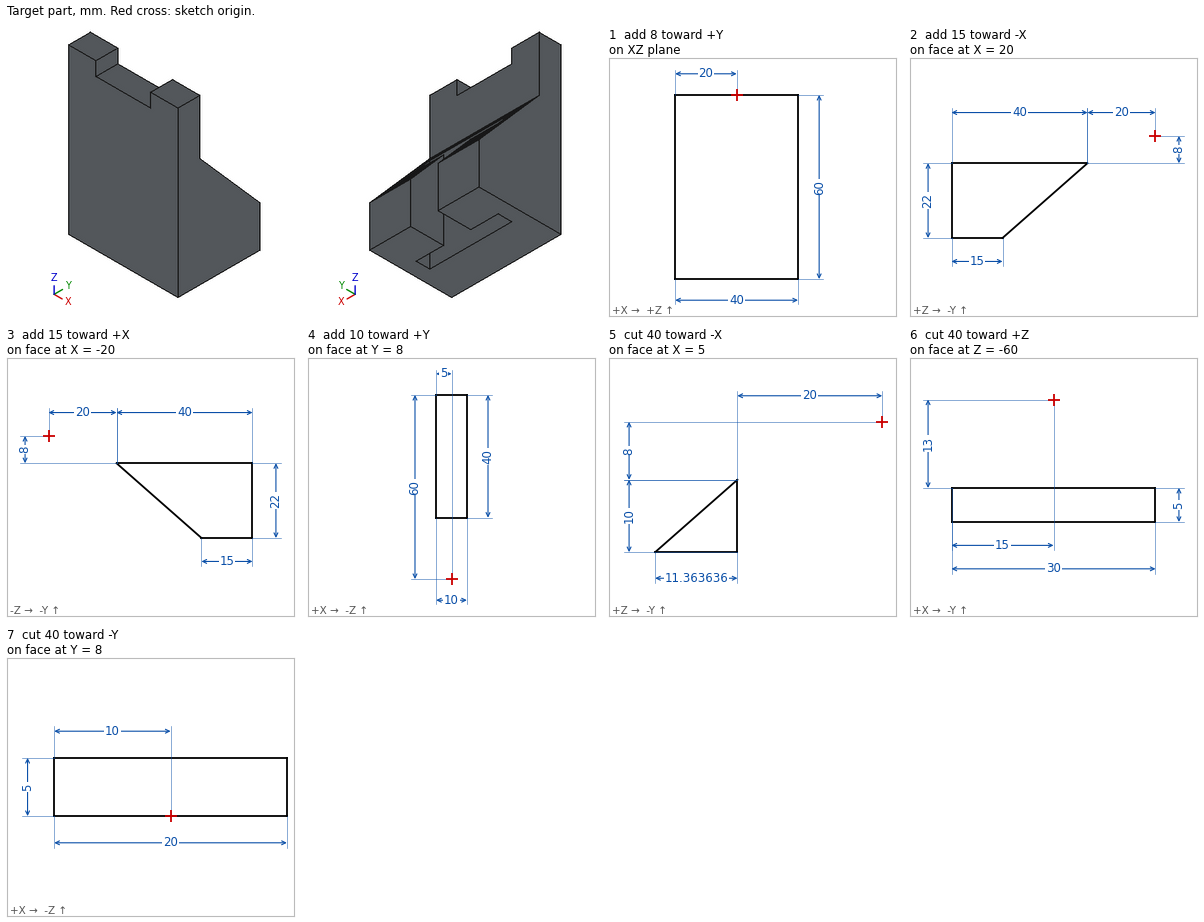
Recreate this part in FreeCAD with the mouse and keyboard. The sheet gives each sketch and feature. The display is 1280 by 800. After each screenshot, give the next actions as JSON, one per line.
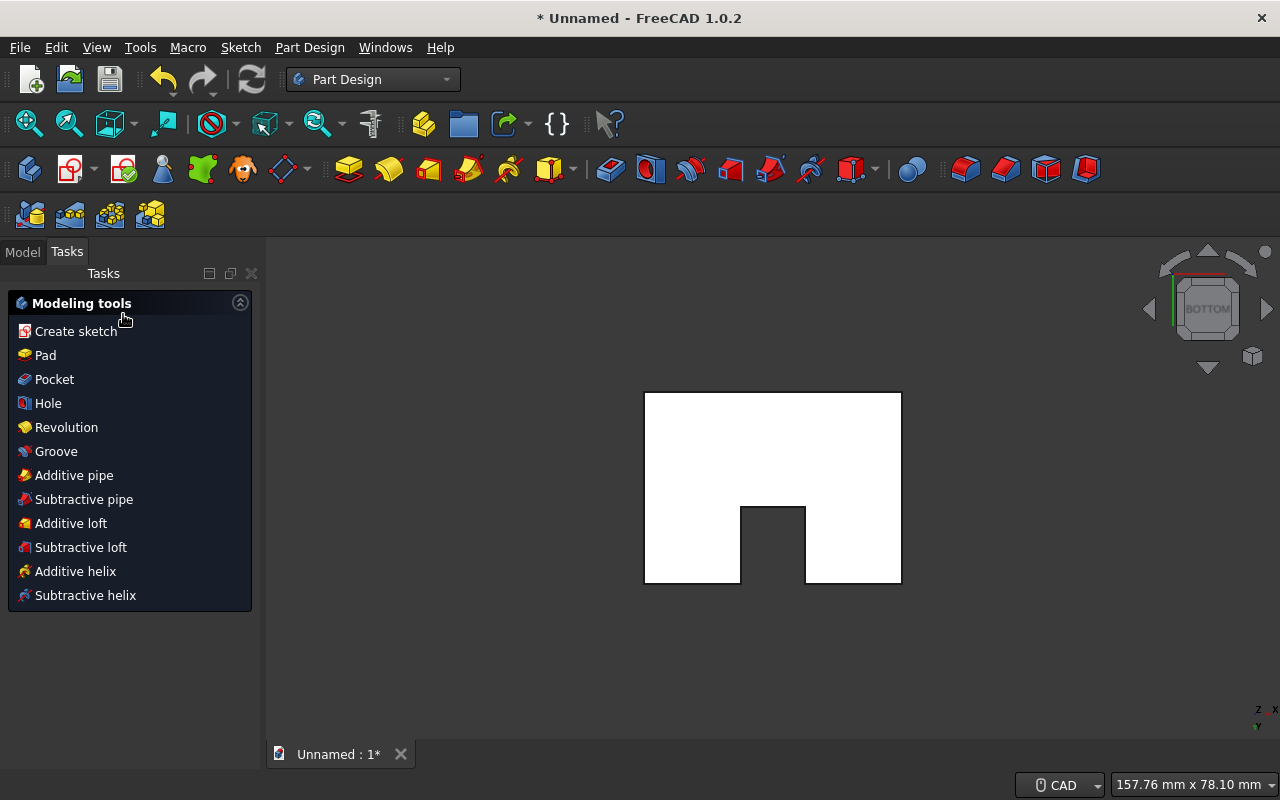
{"action": "left_click", "coordinate": [612, 170]}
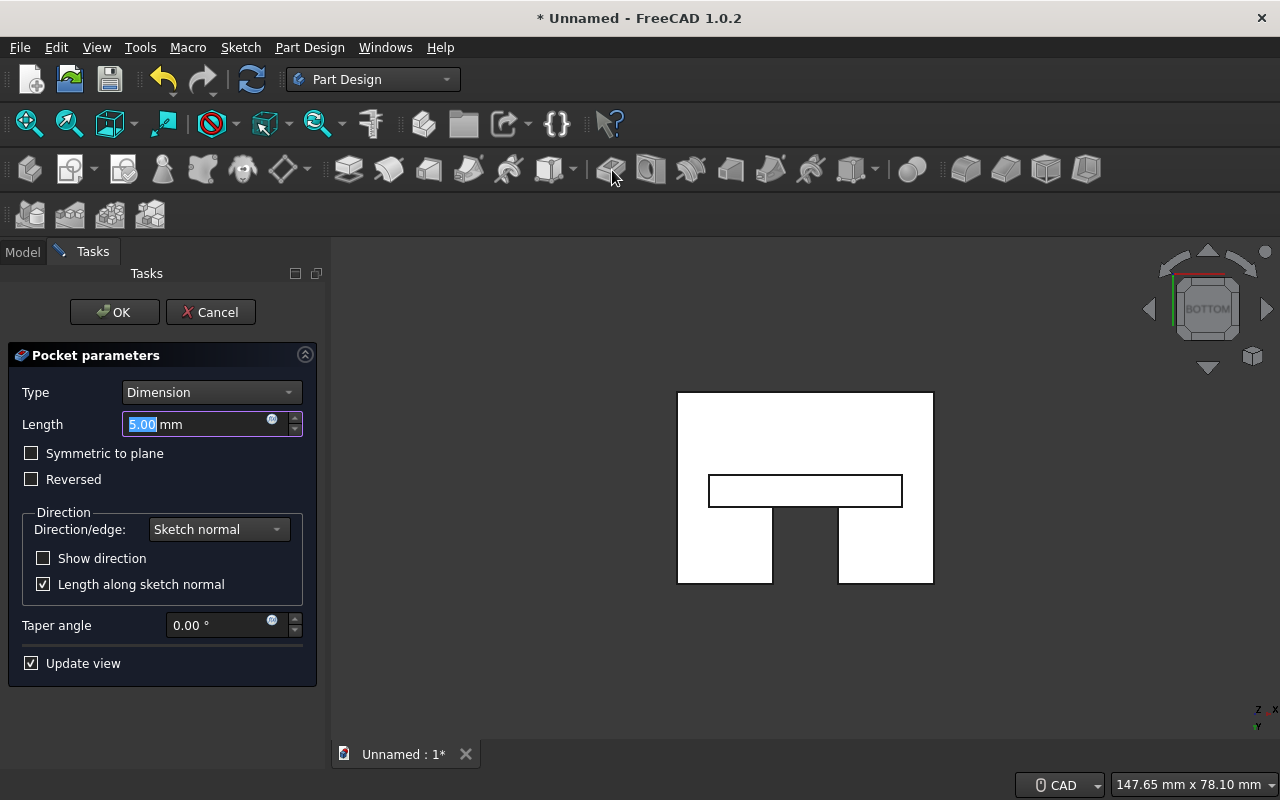
{"action": "type", "text": "40"}
{"action": "key", "text": "Tab"}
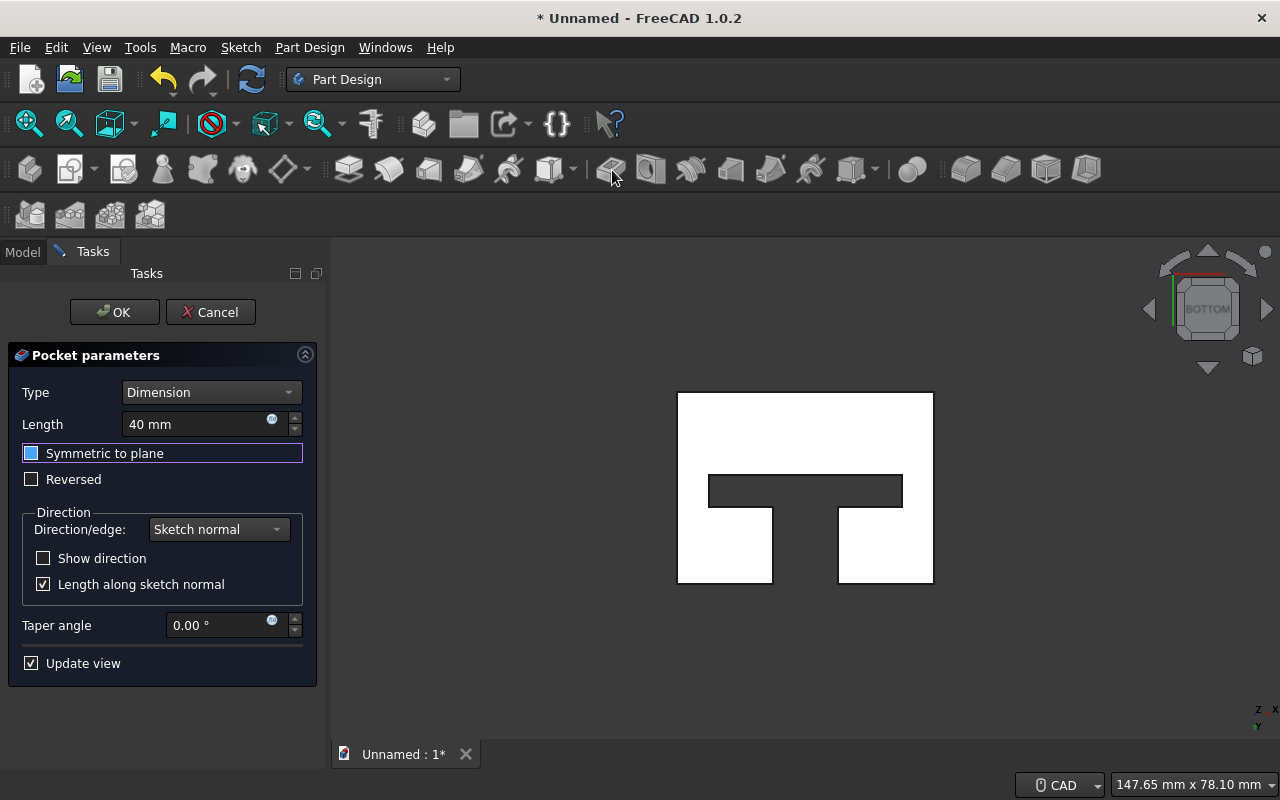
{"action": "left_click", "coordinate": [115, 312]}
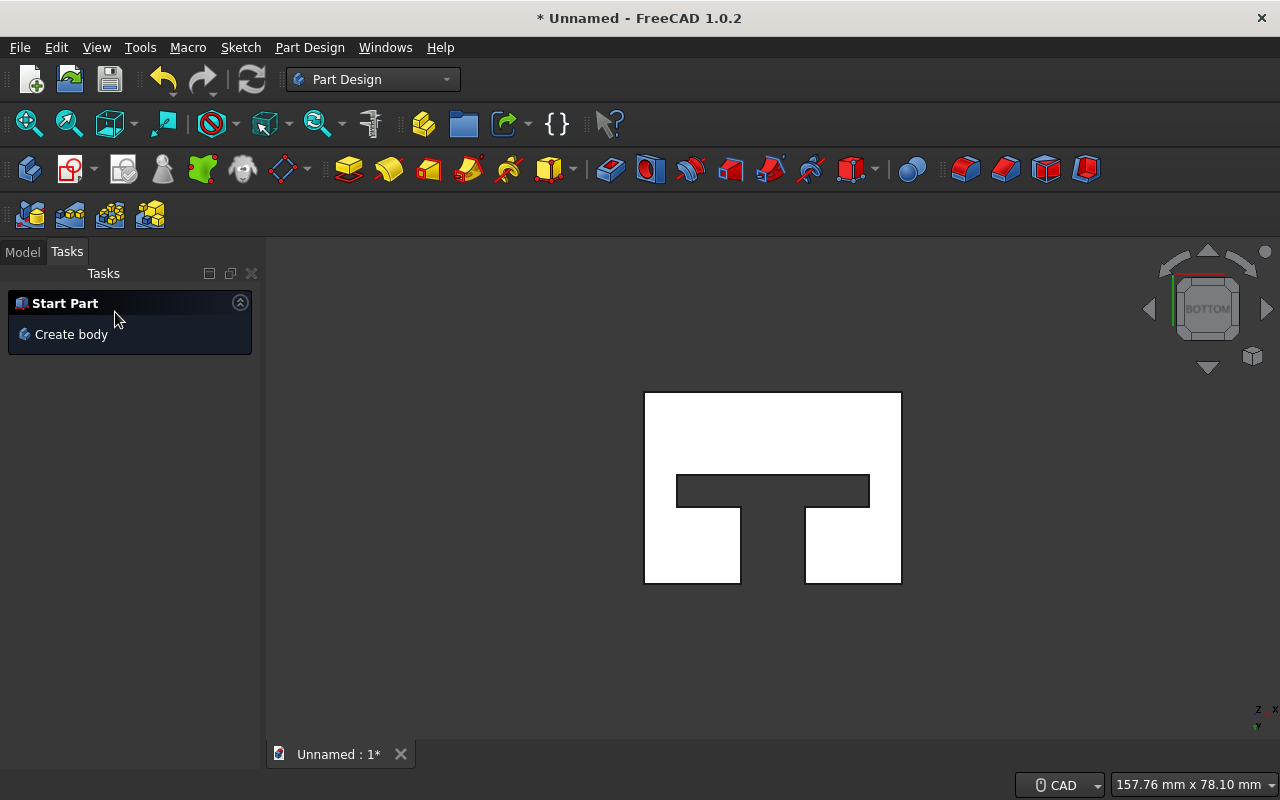
{"action": "left_click", "coordinate": [30, 124]}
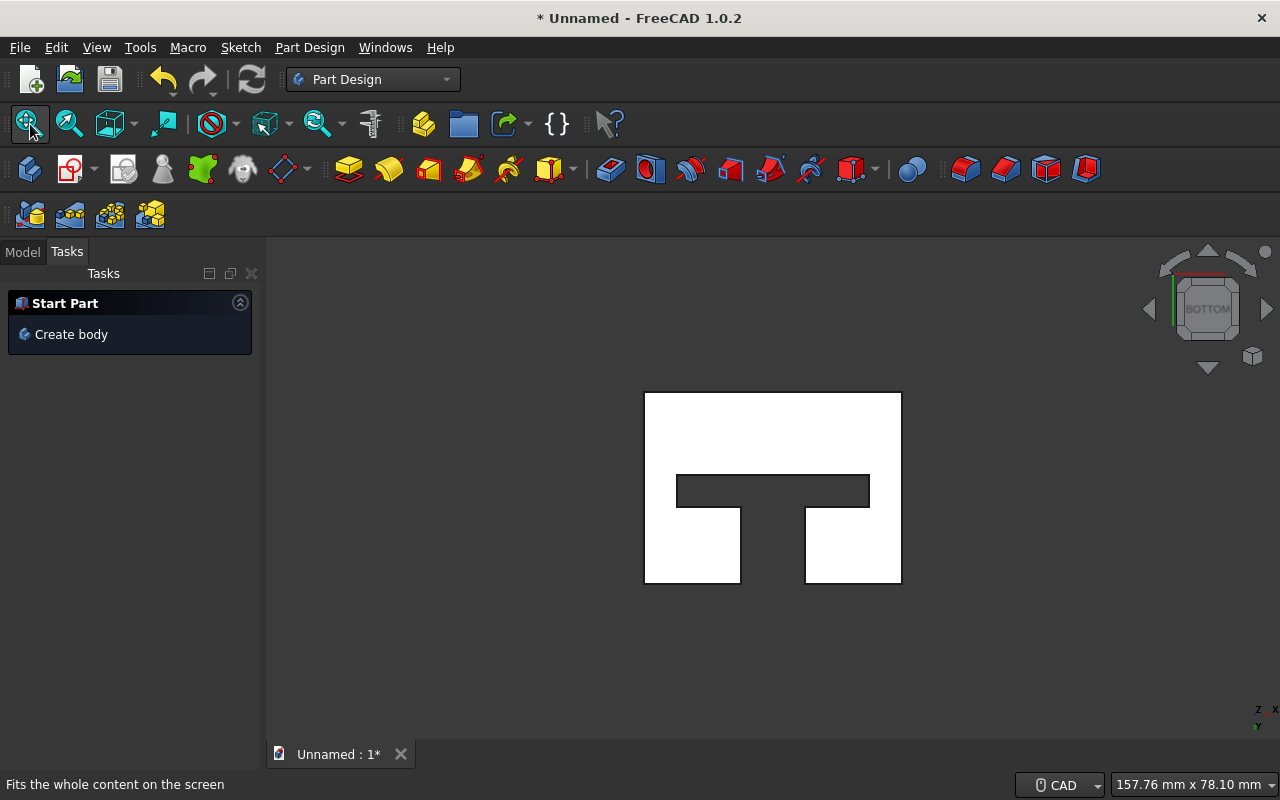
{"action": "key", "text": "4"}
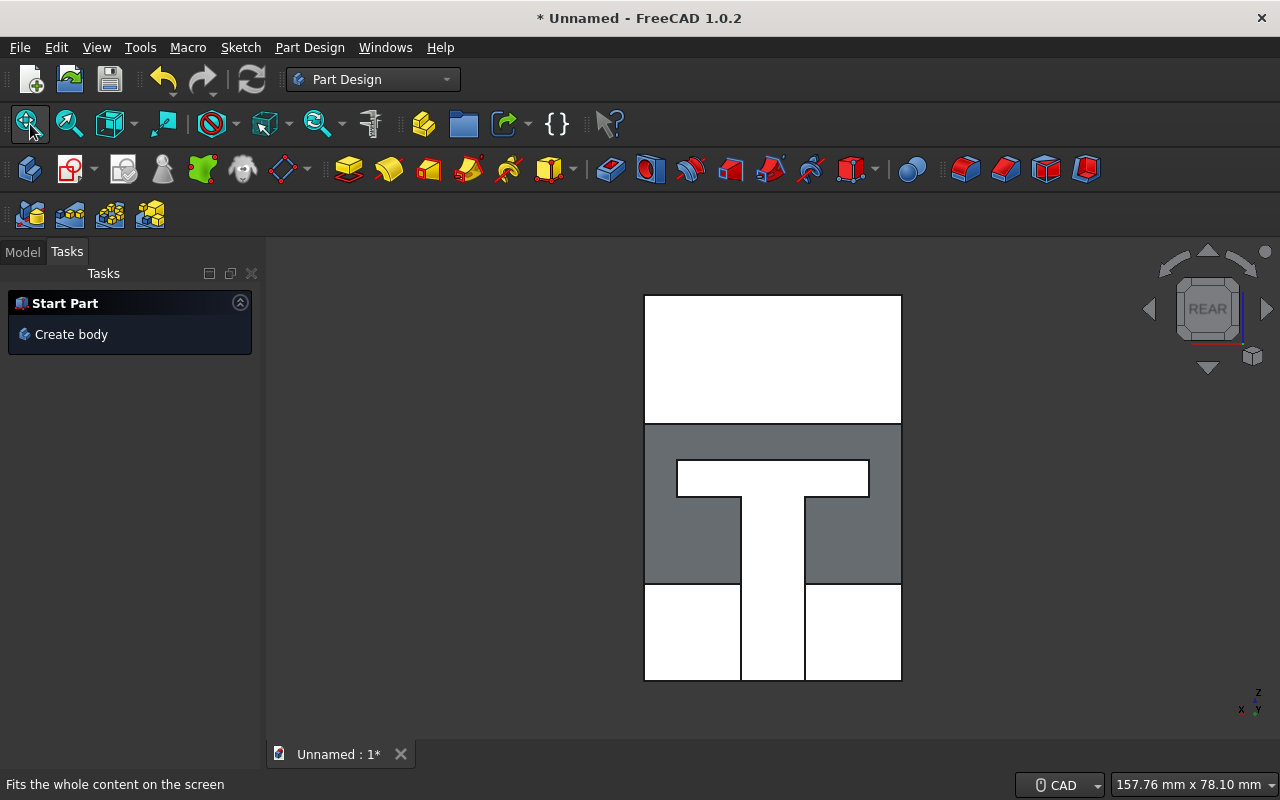
{"action": "left_click", "coordinate": [736, 358]}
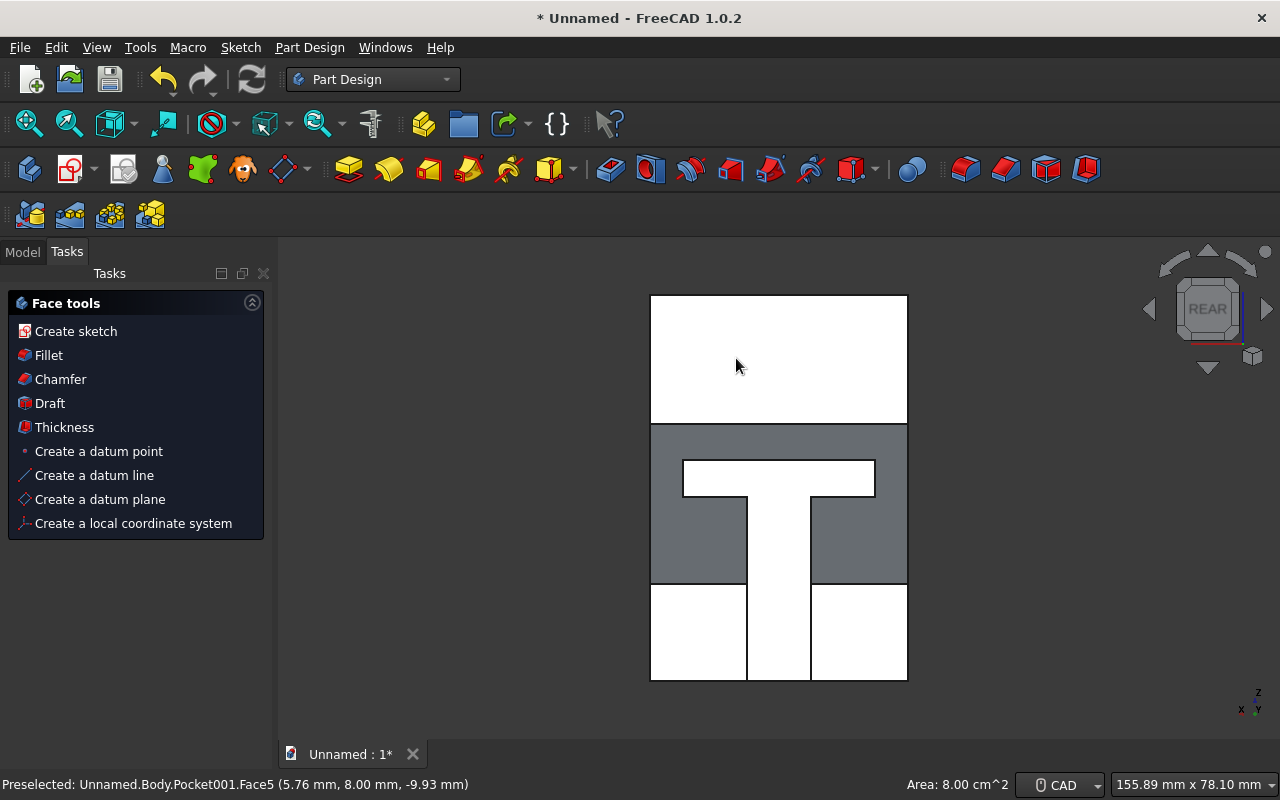
{"action": "left_click", "coordinate": [70, 170]}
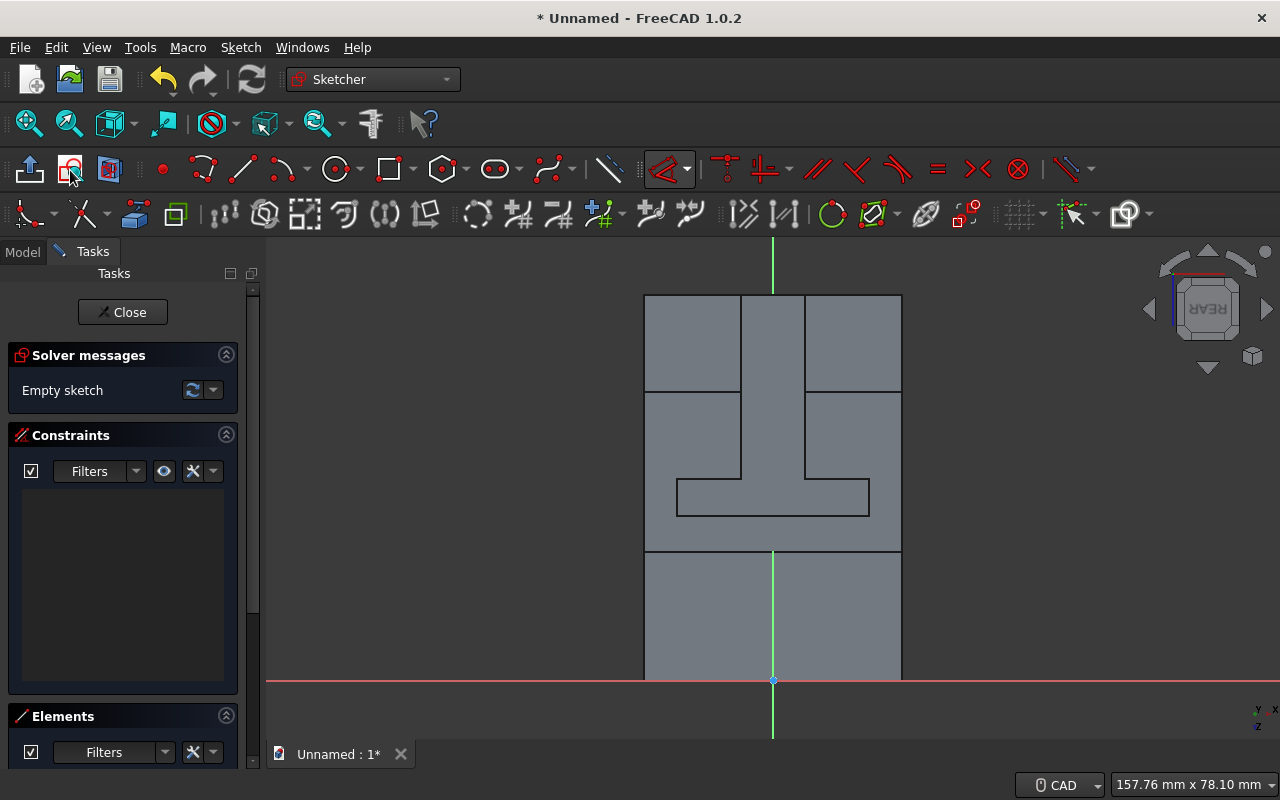
{"action": "left_click", "coordinate": [110, 170]}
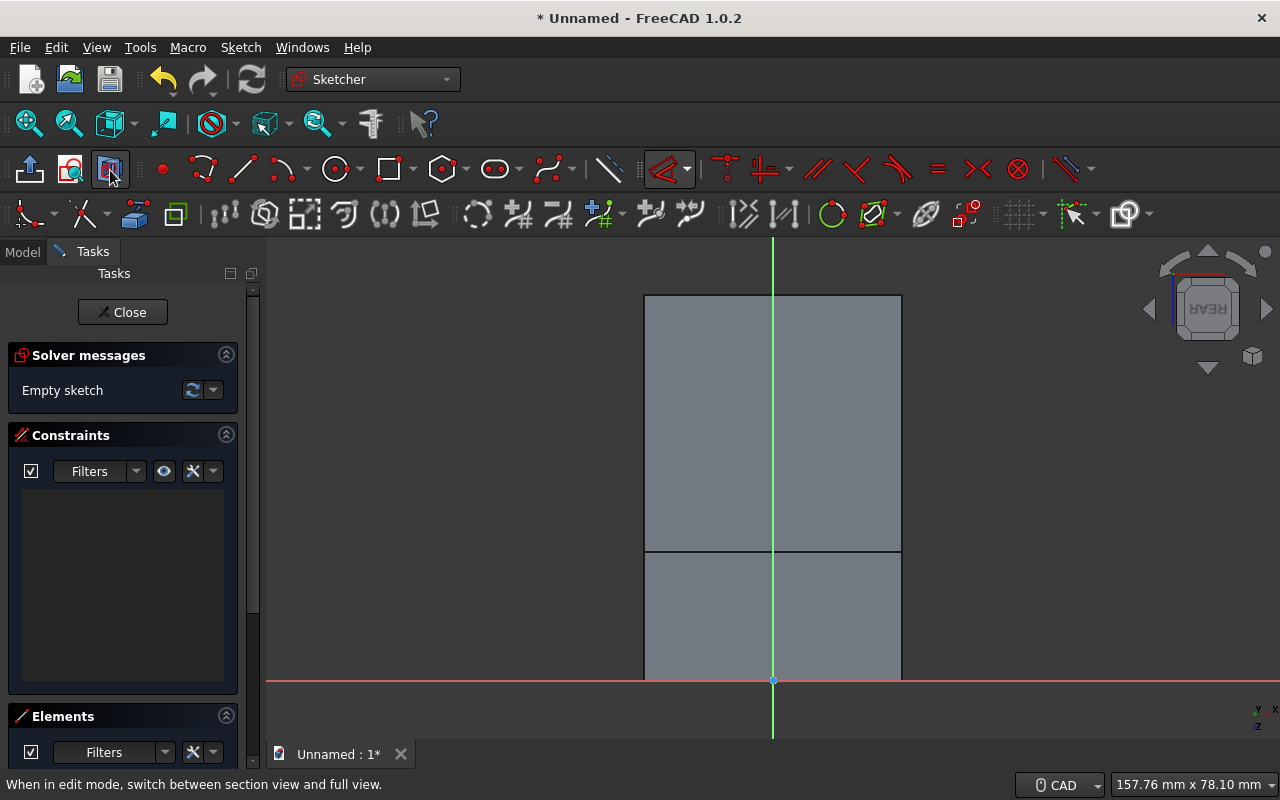
{"action": "scroll", "coordinate": [790, 709], "scroll_direction": "up", "scroll_amount": 8}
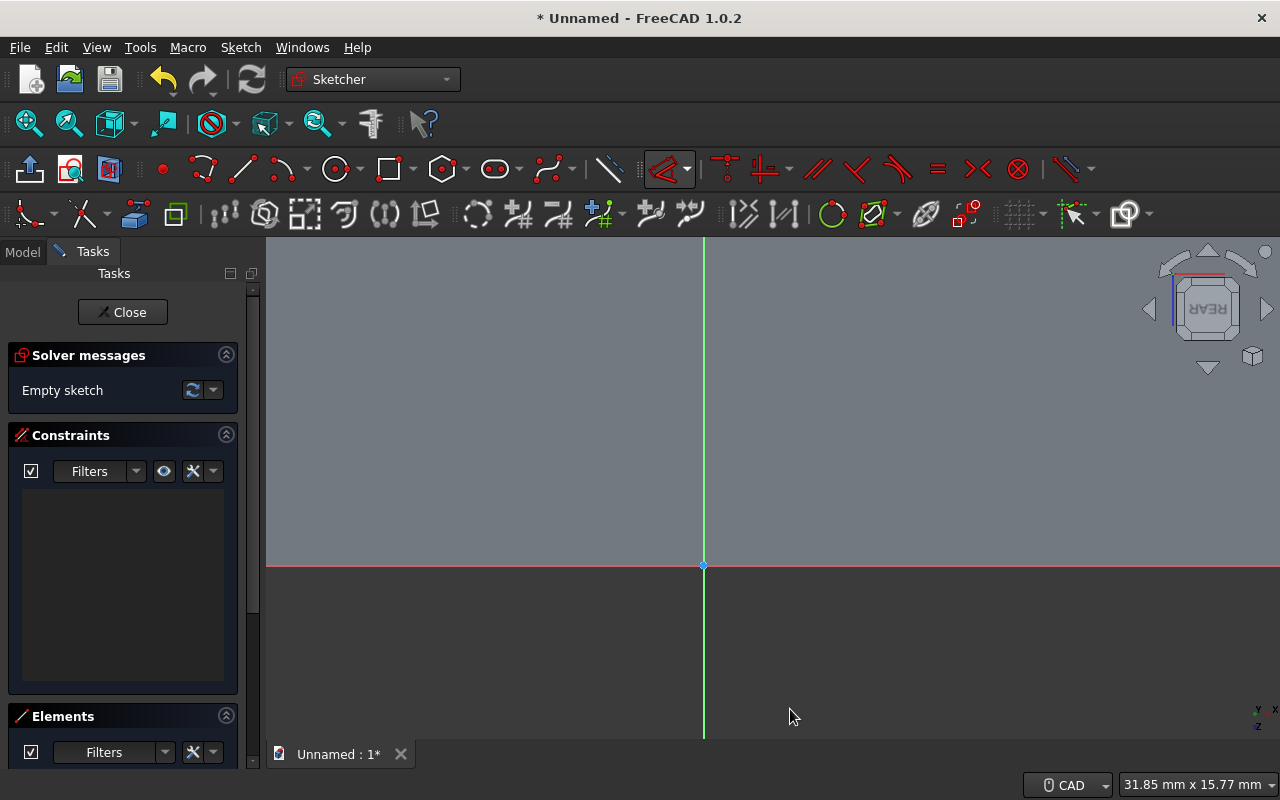
{"action": "left_click", "coordinate": [390, 170]}